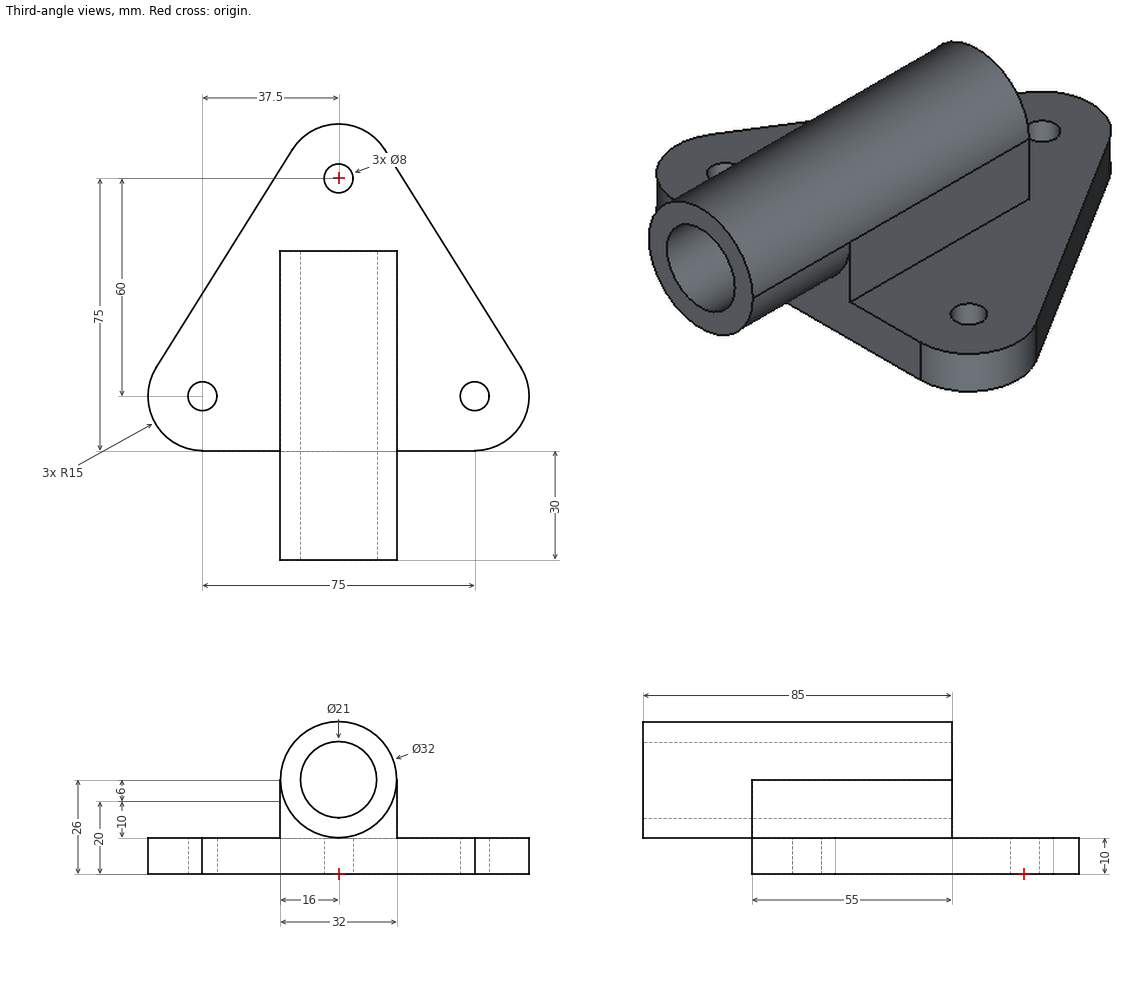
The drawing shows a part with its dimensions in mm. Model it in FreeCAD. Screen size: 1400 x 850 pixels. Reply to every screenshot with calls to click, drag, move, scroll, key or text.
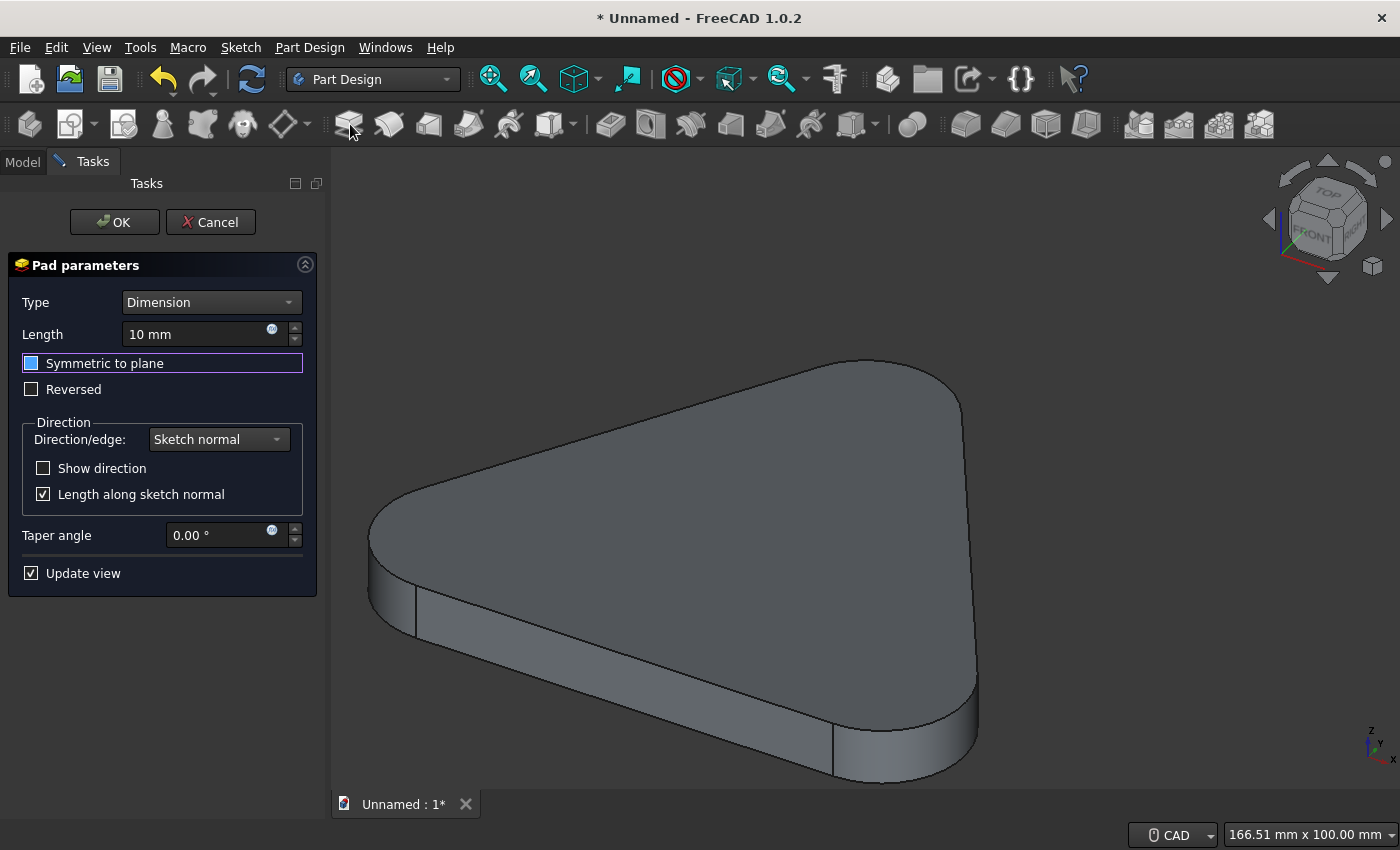
click(115, 222)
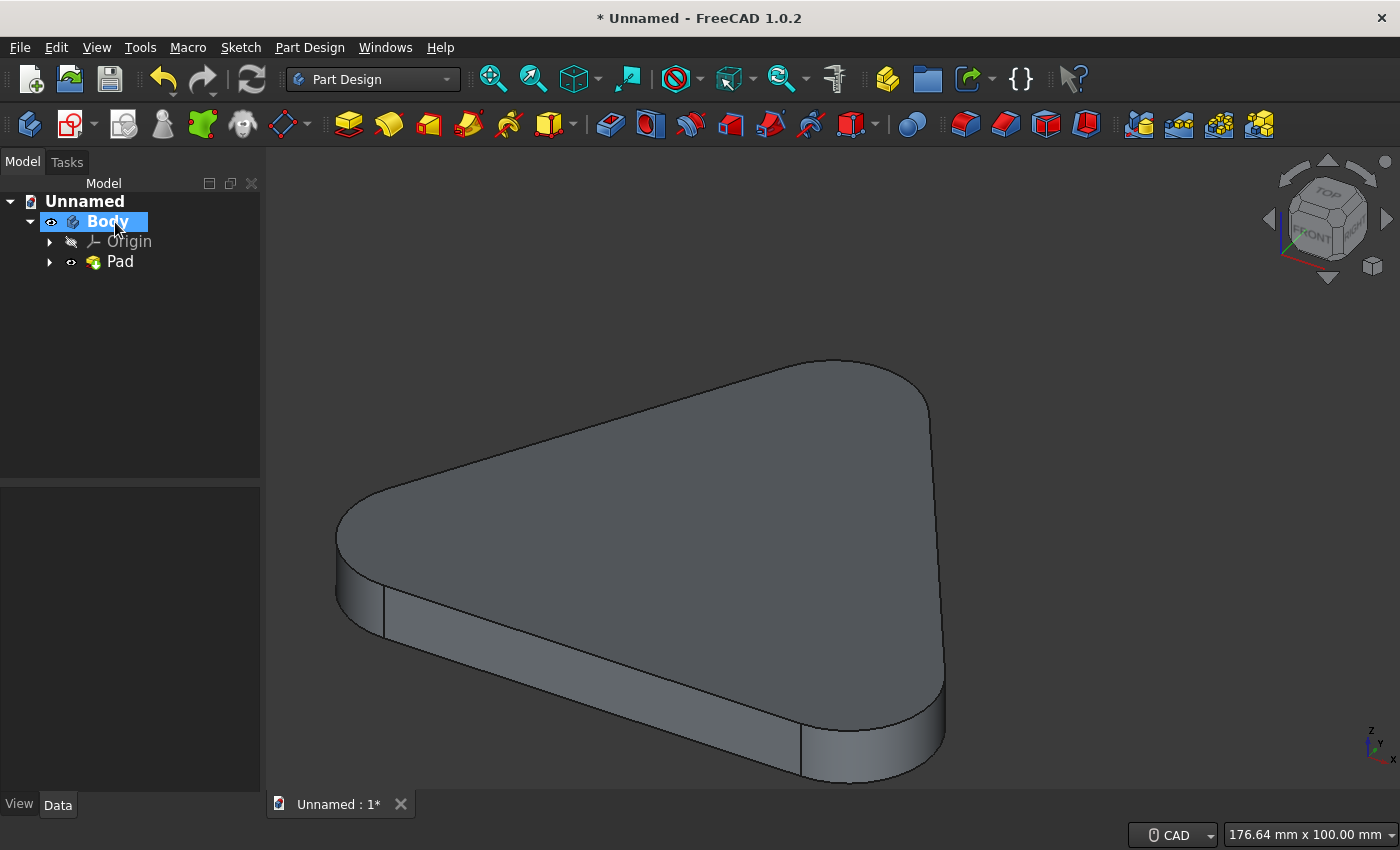
click(494, 80)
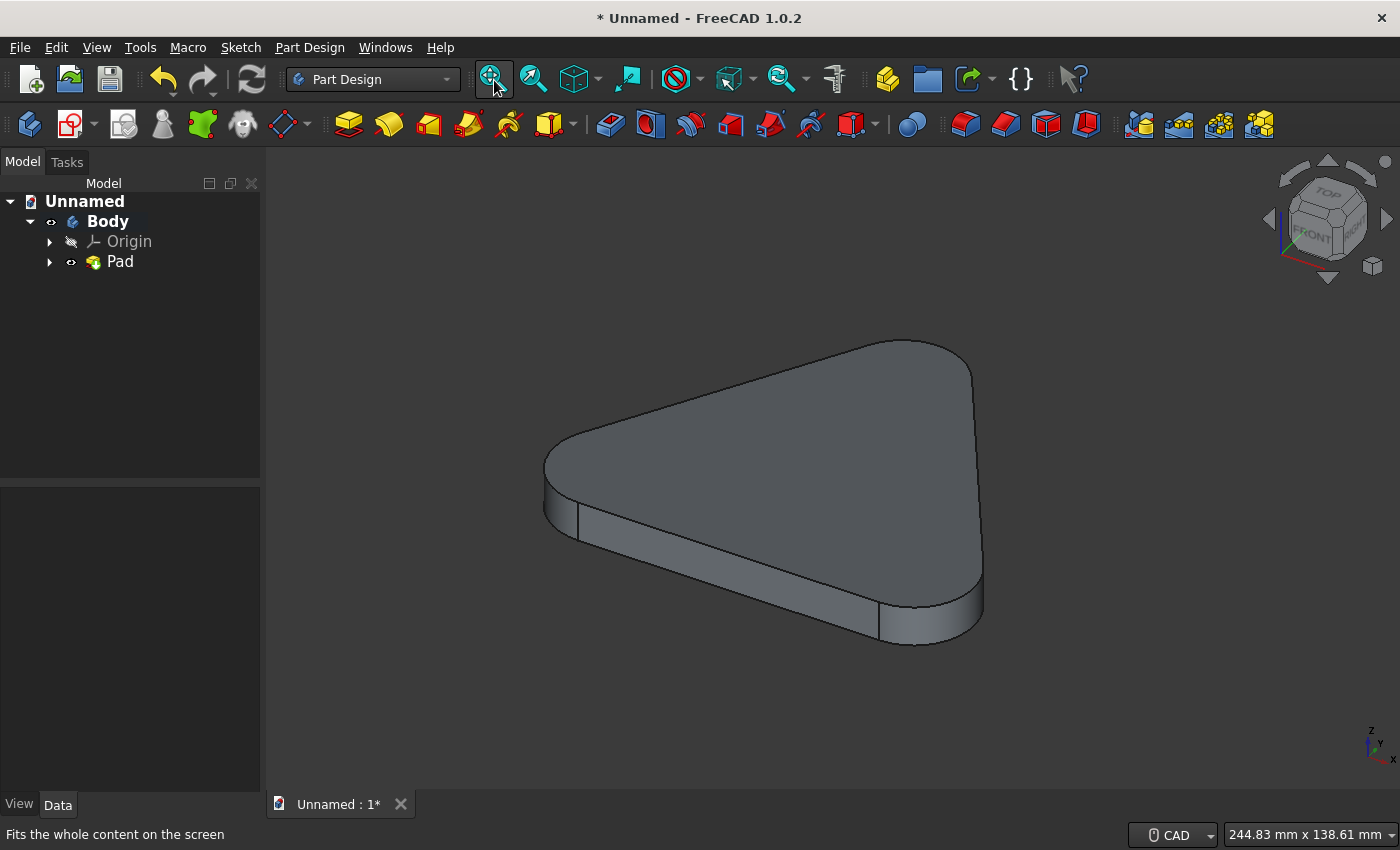
click(858, 613)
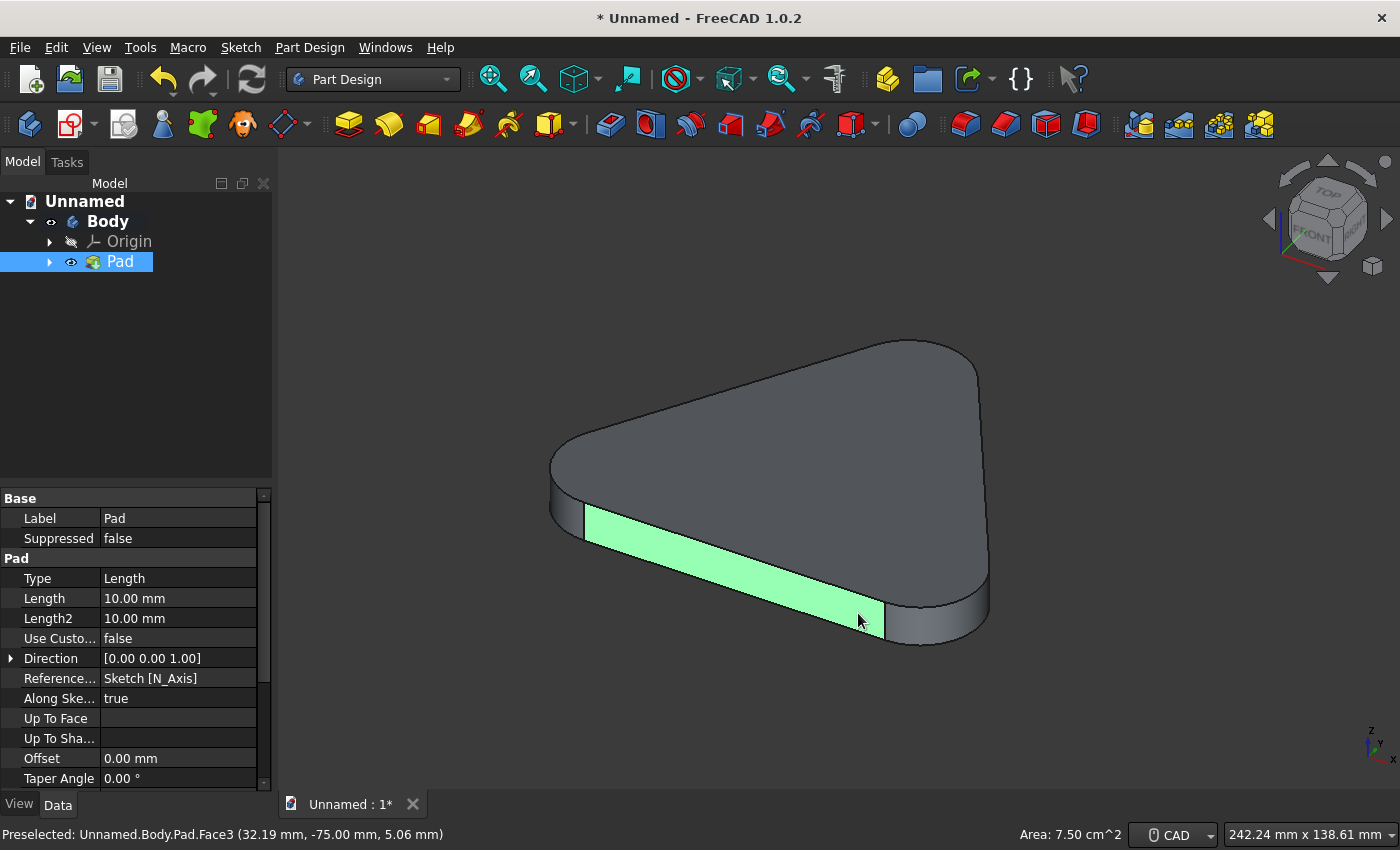
click(70, 124)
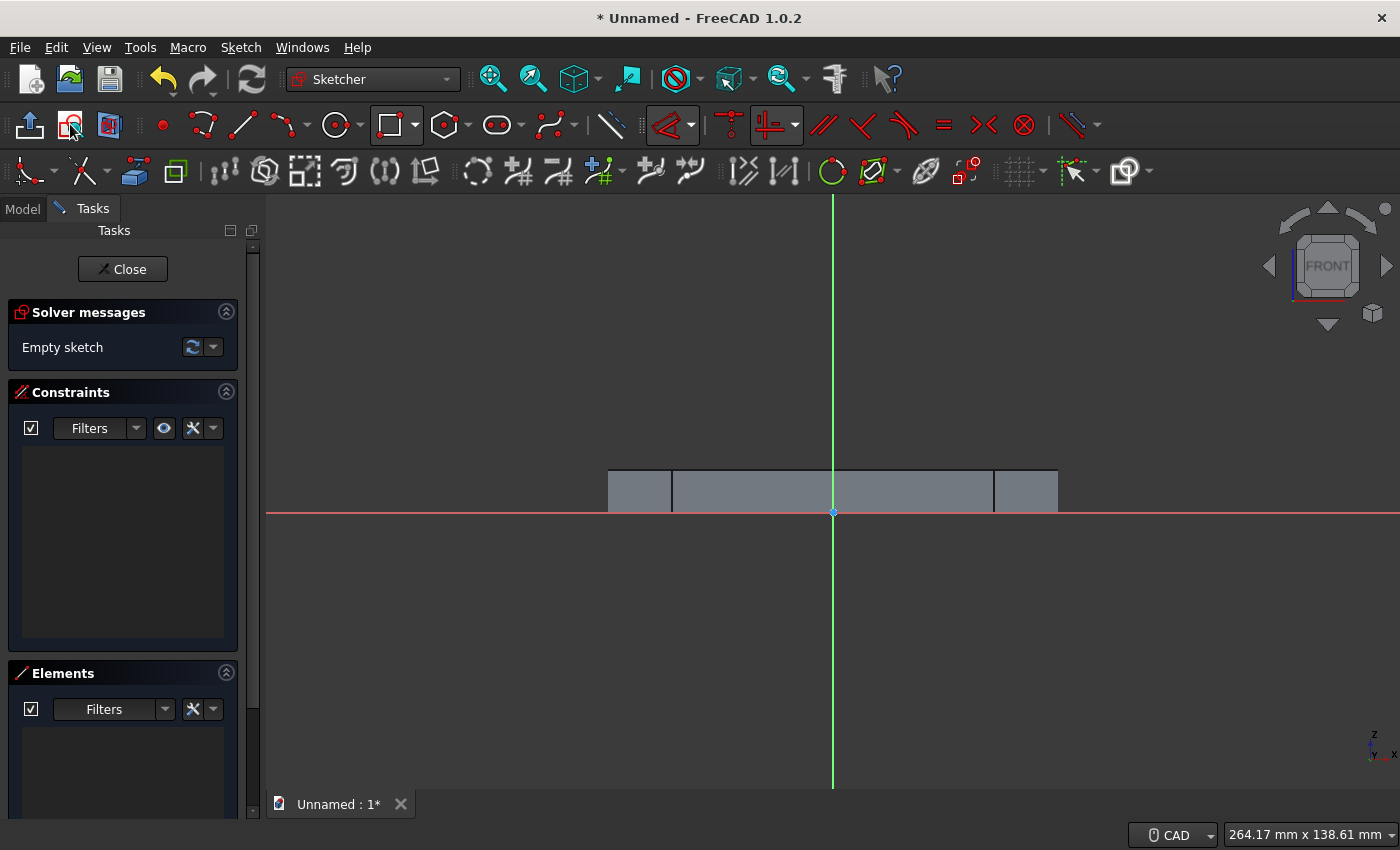
scroll(855, 463, up, 7)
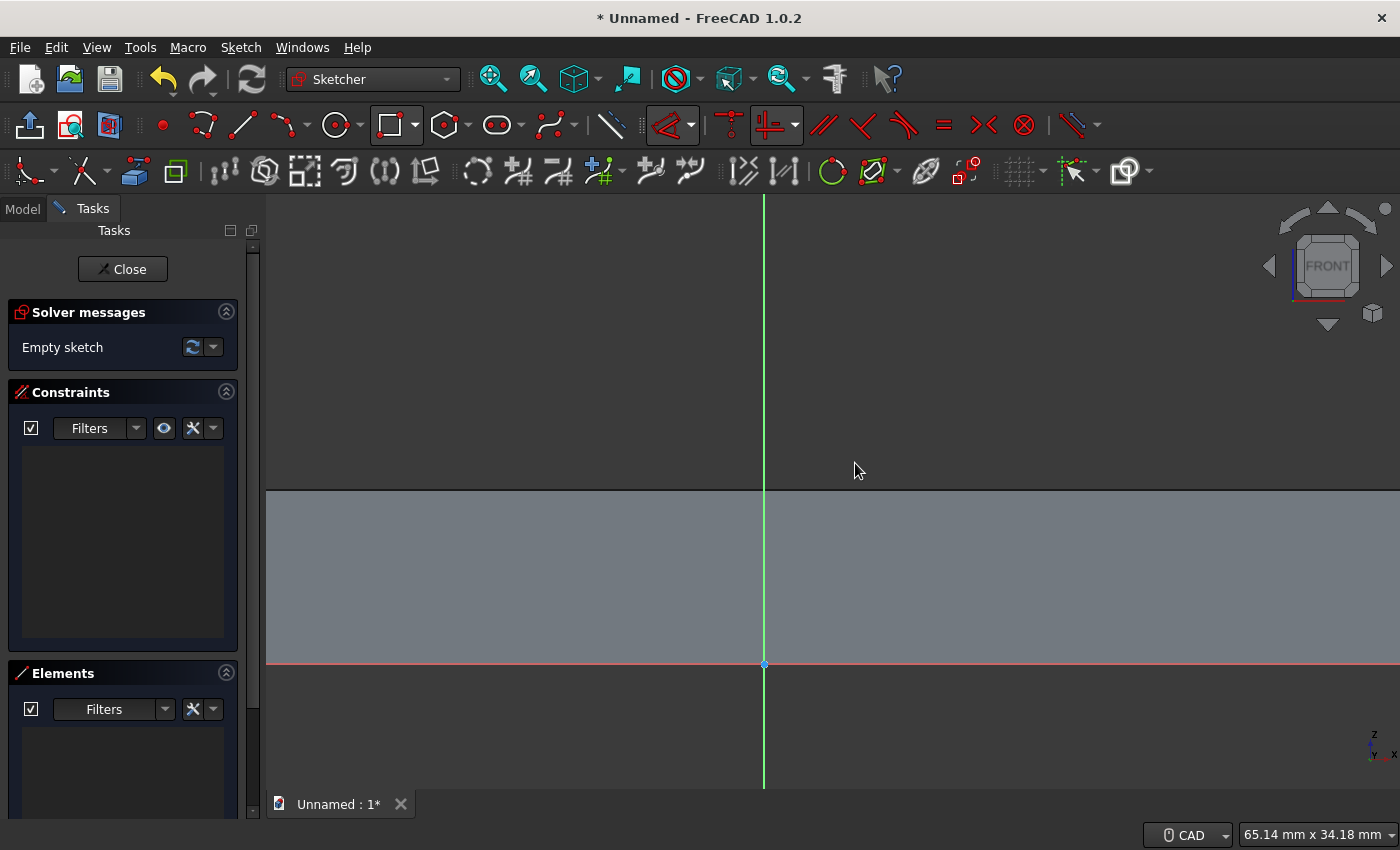
click(390, 126)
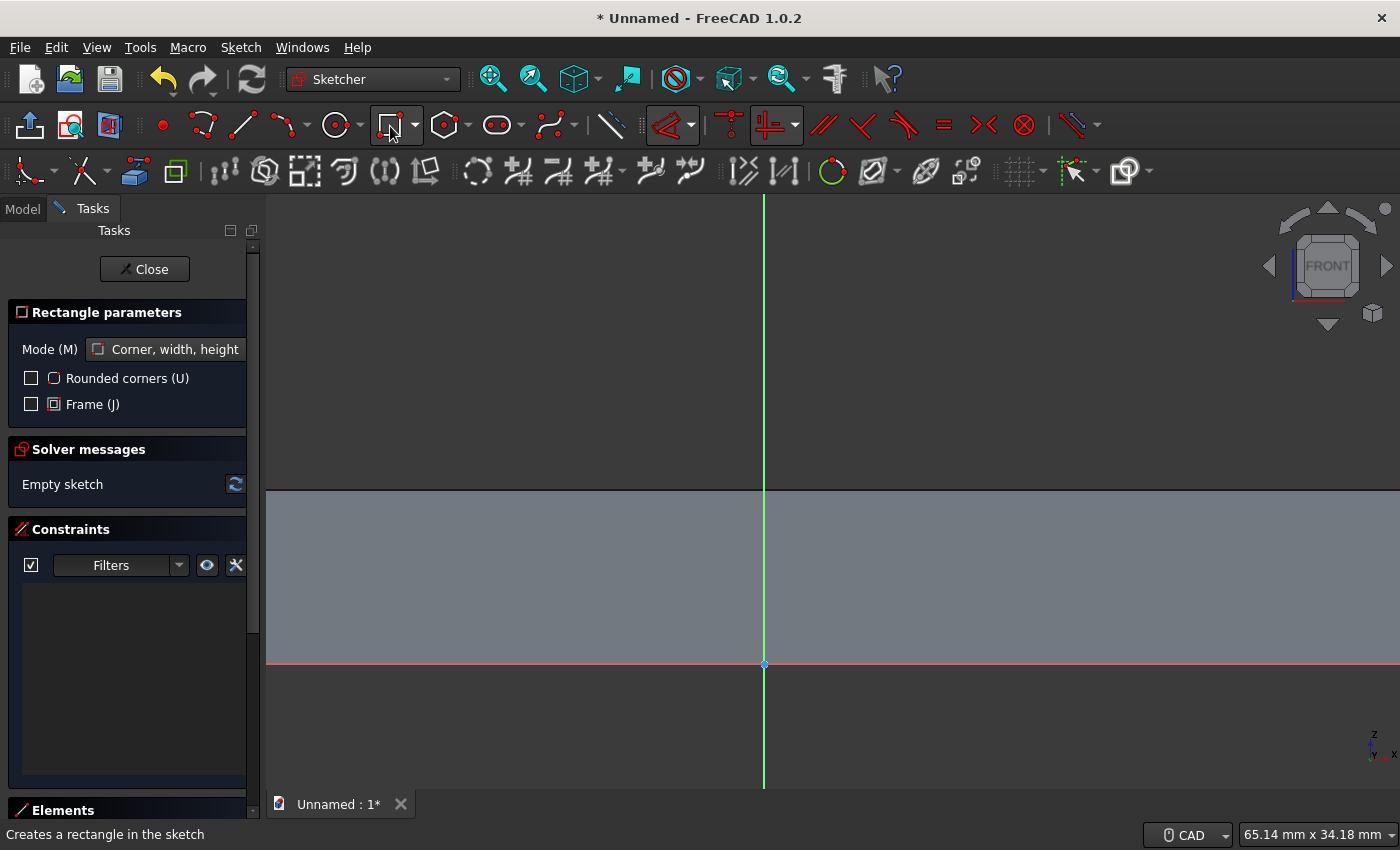
click(486, 316)
click(1043, 490)
key(Escape)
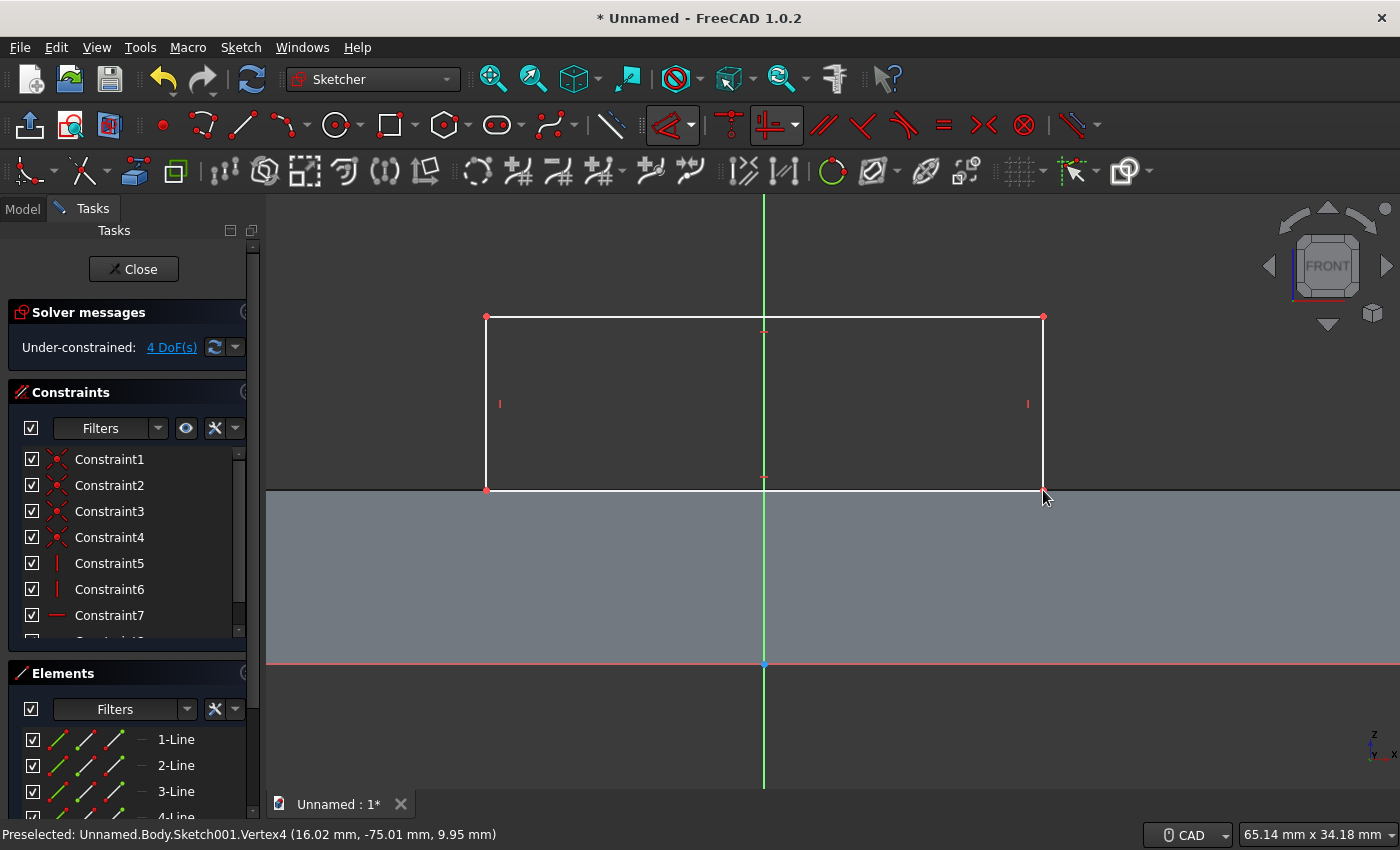
click(486, 369)